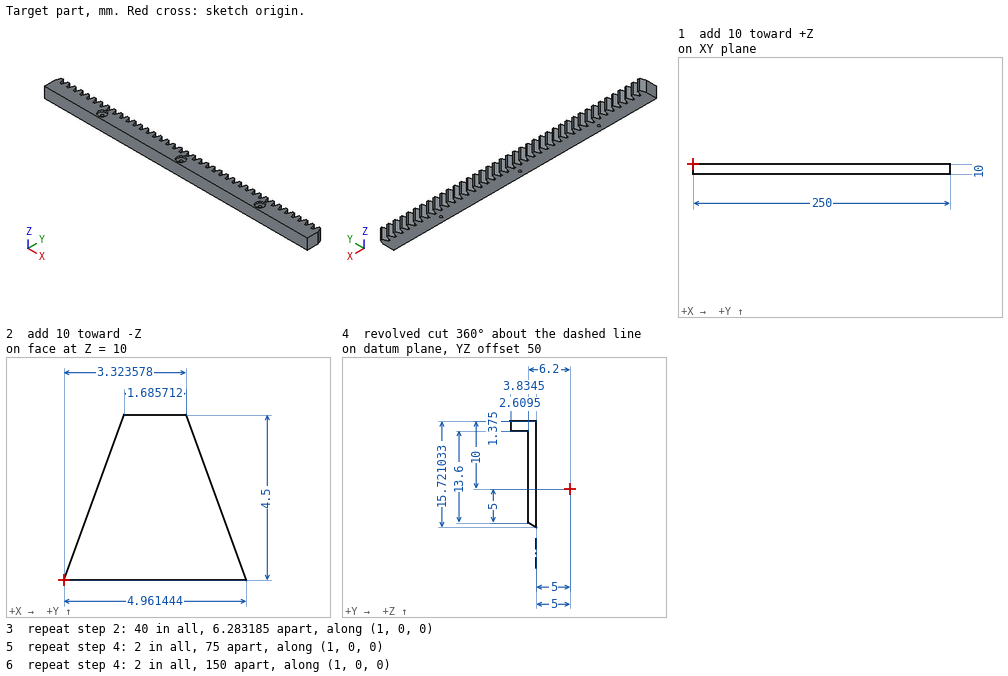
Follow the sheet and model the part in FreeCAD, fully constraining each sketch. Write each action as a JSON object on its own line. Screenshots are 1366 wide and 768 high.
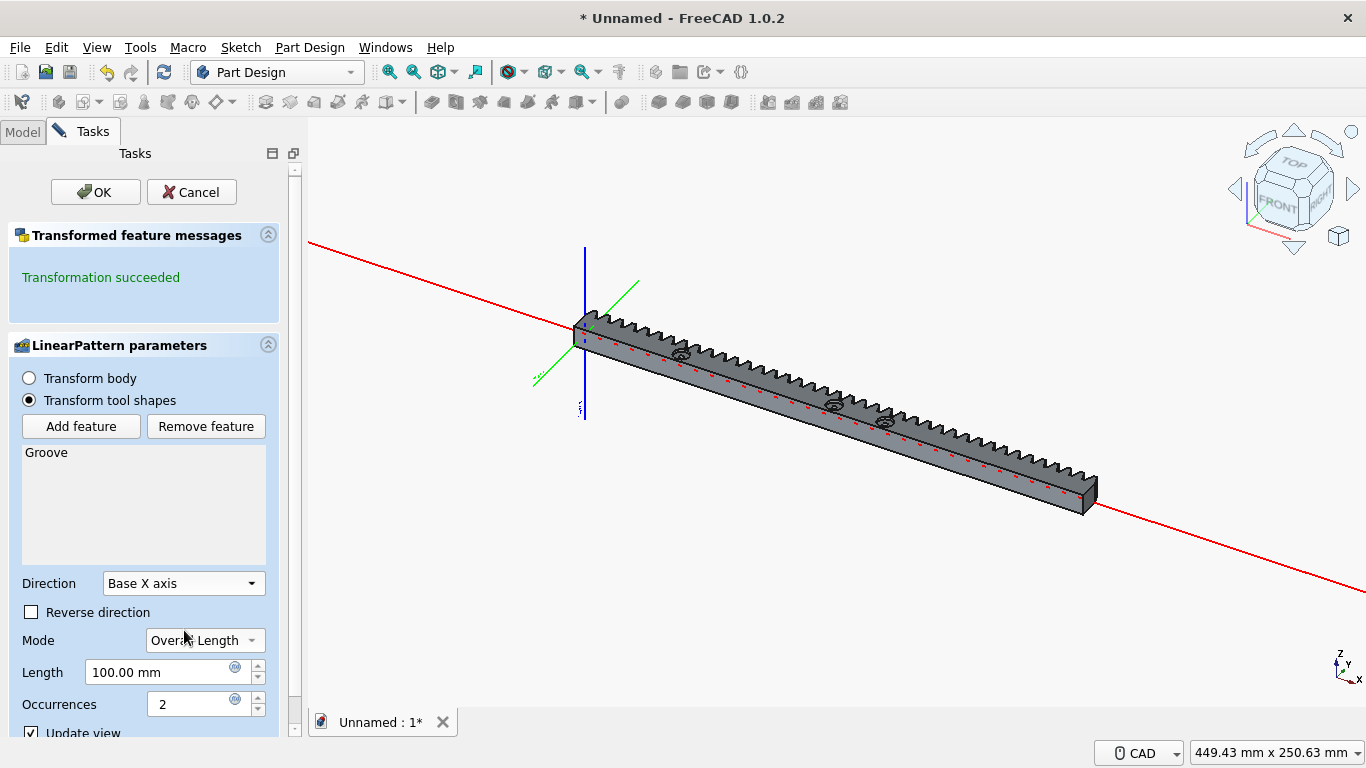
{"action": "left_click", "coordinate": [206, 640]}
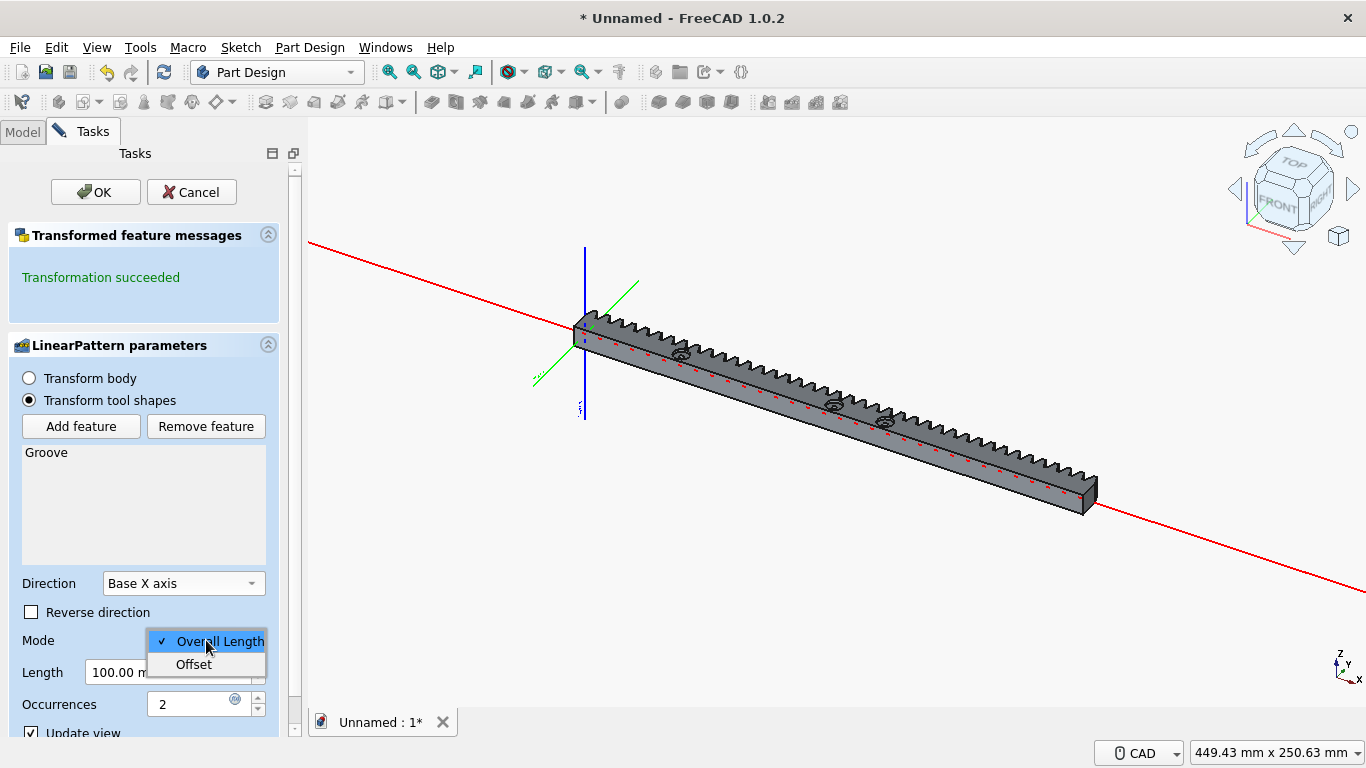
{"action": "left_click", "coordinate": [206, 664]}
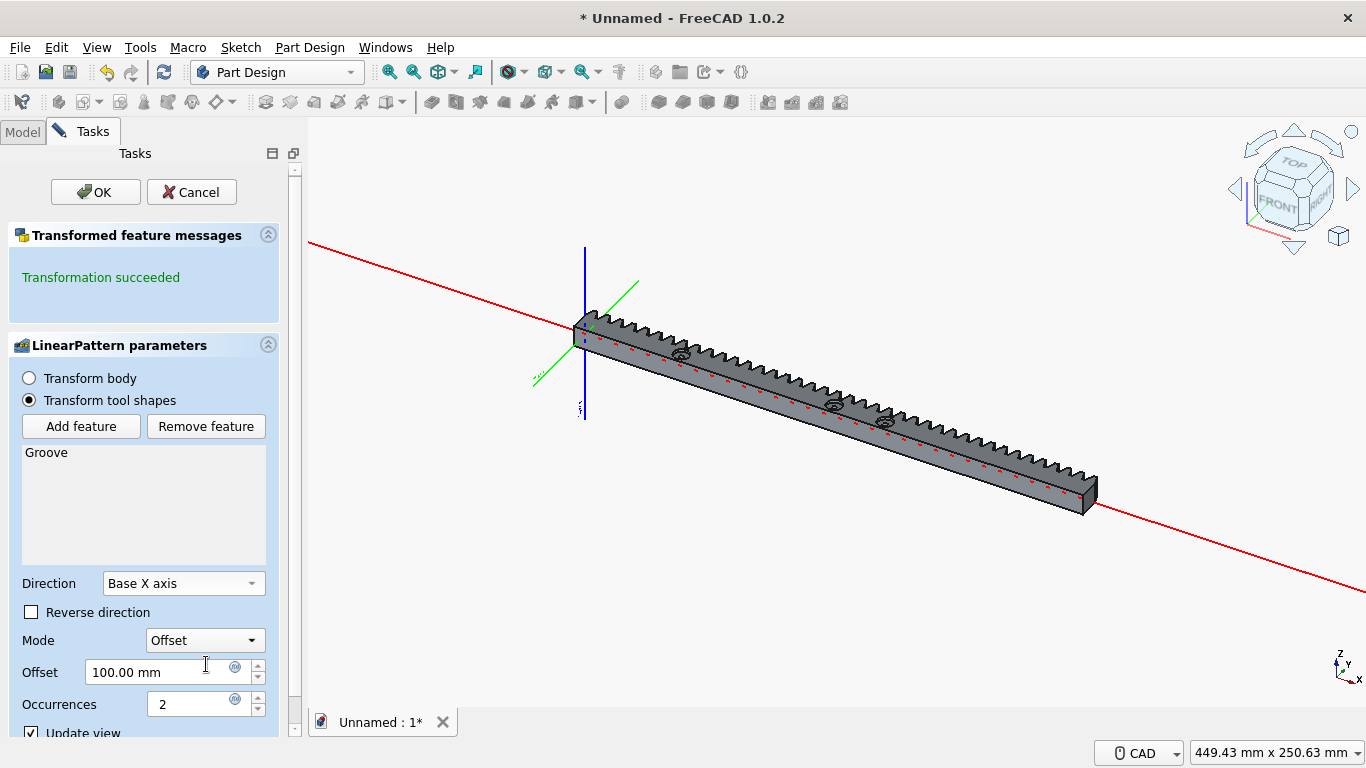
{"action": "triple_click", "coordinate": [168, 672]}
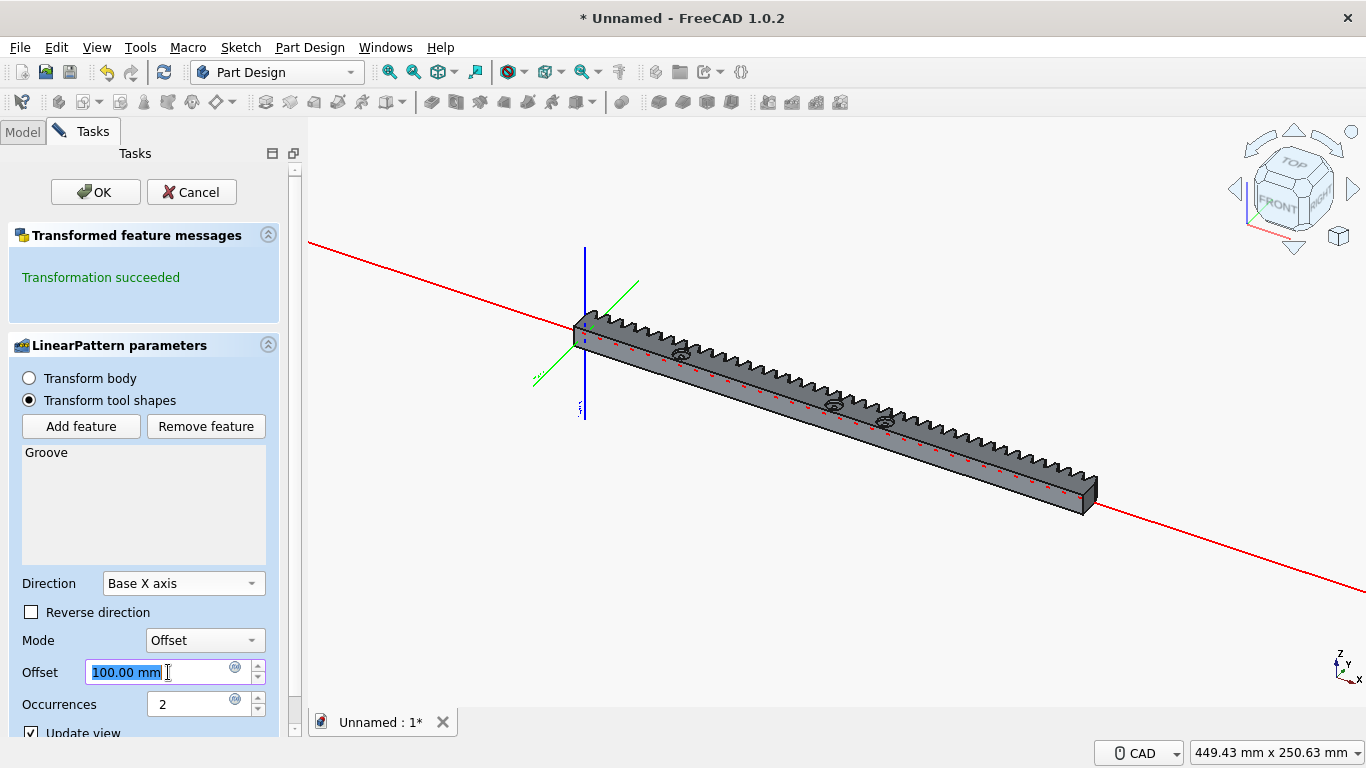
{"action": "type", "text": "150"}
{"action": "key", "text": "Tab"}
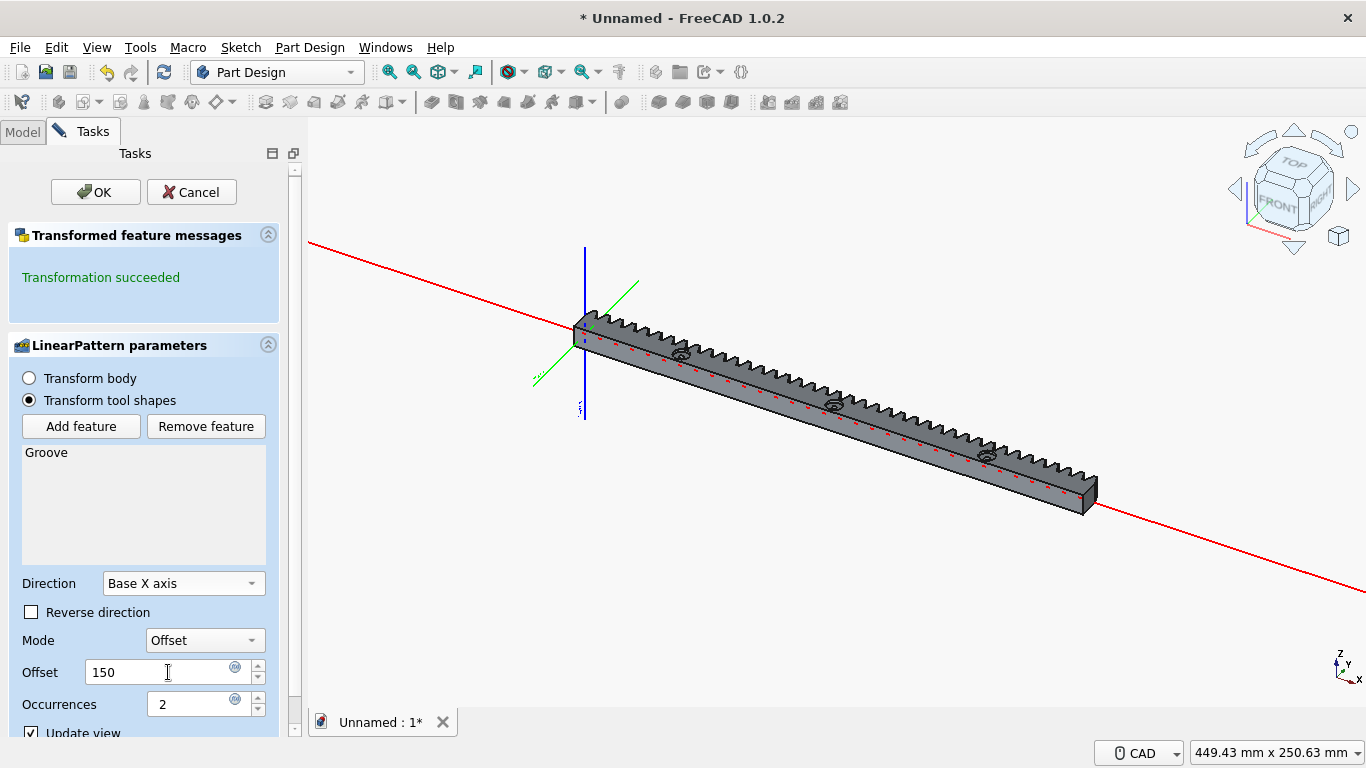
{"action": "triple_click", "coordinate": [198, 704]}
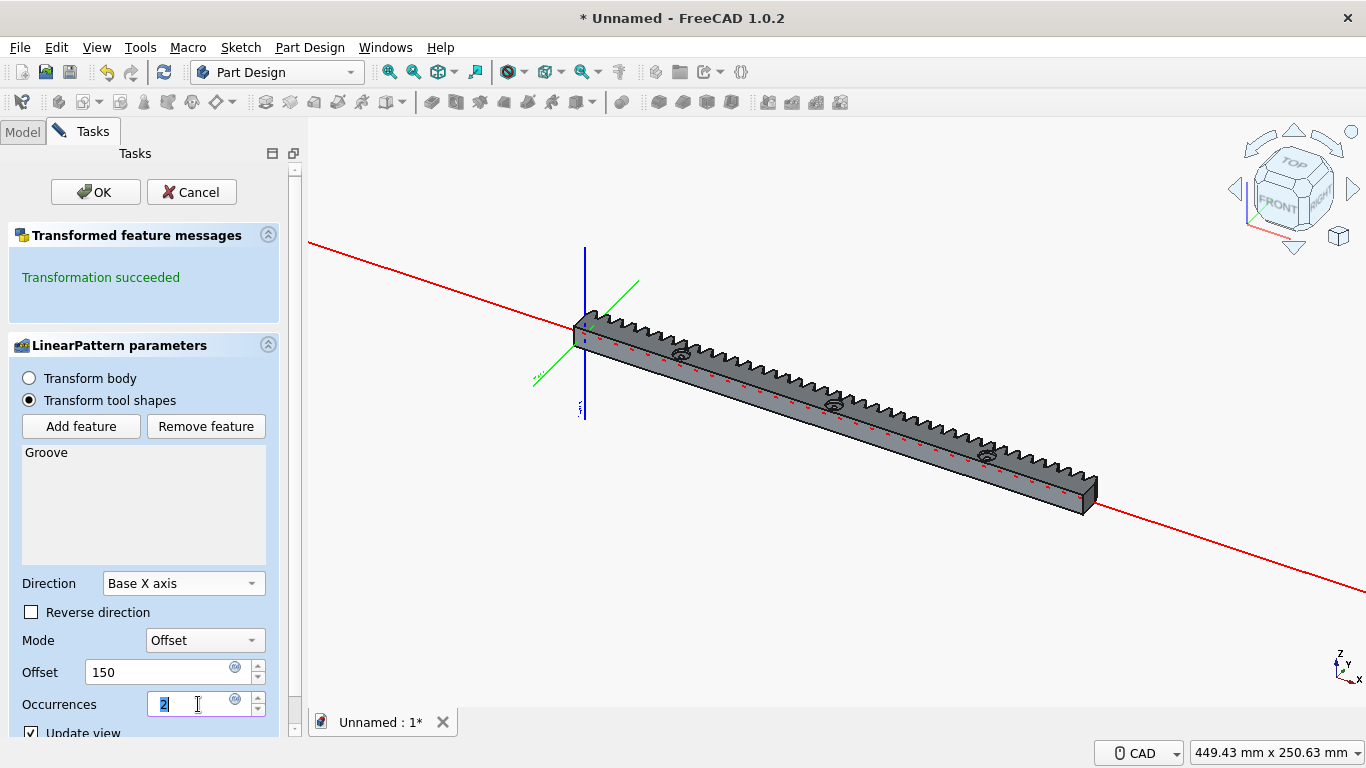
{"action": "type", "text": "2"}
{"action": "key", "text": "Tab"}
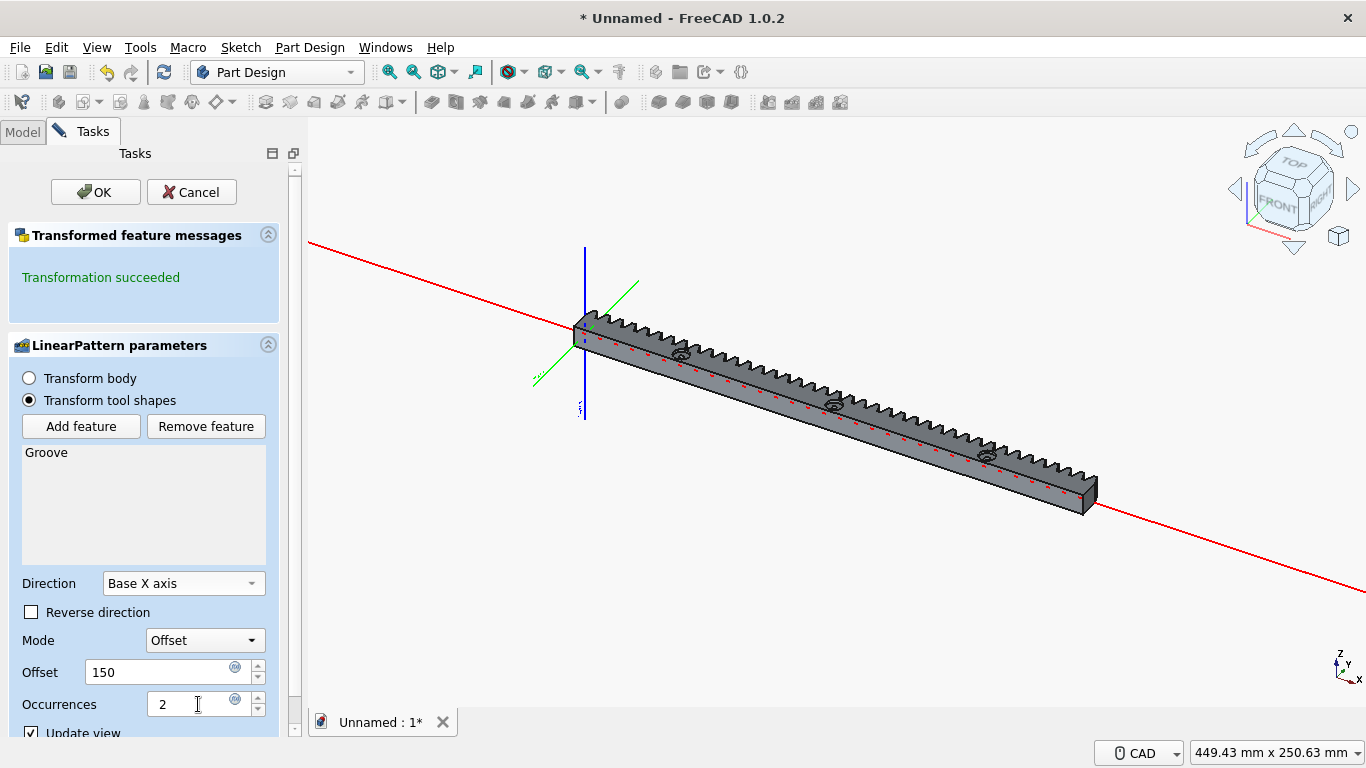
{"action": "left_click", "coordinate": [96, 192]}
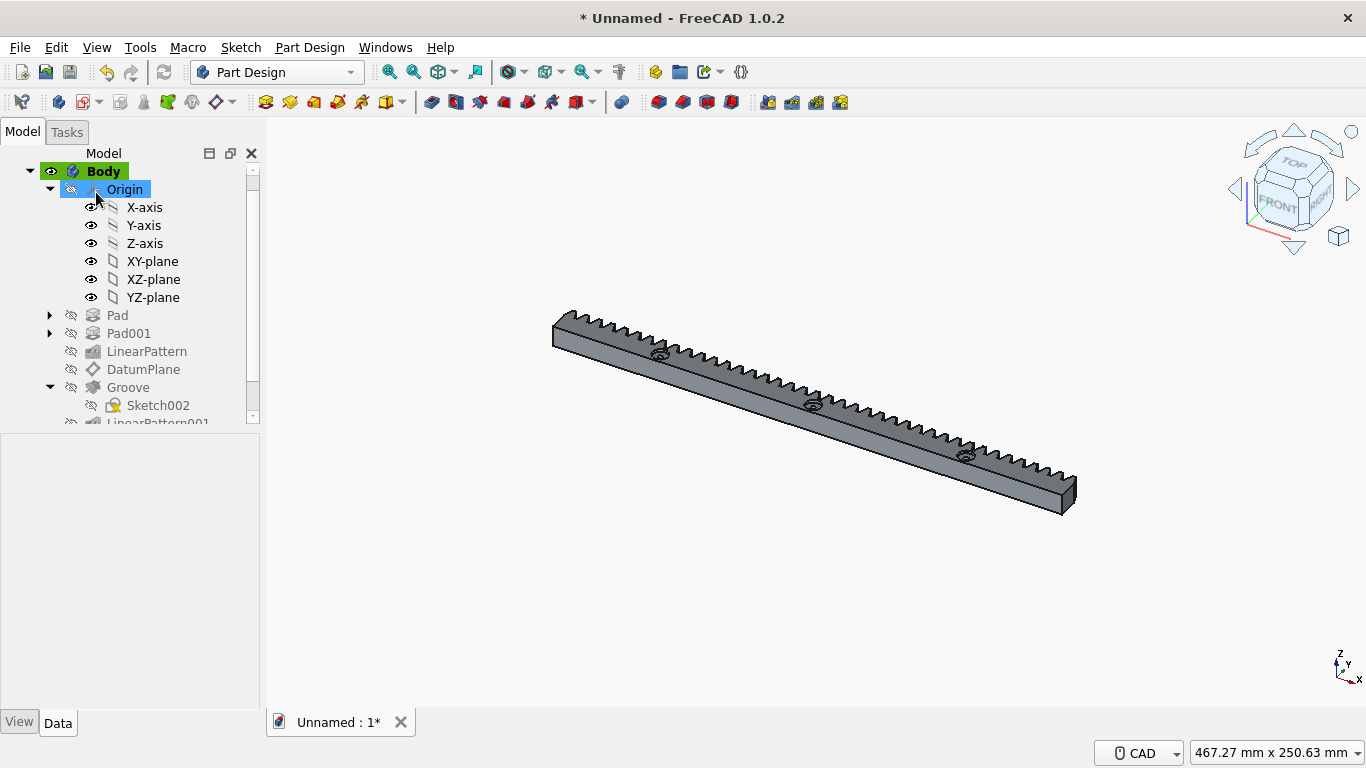
{"action": "key", "text": "0"}